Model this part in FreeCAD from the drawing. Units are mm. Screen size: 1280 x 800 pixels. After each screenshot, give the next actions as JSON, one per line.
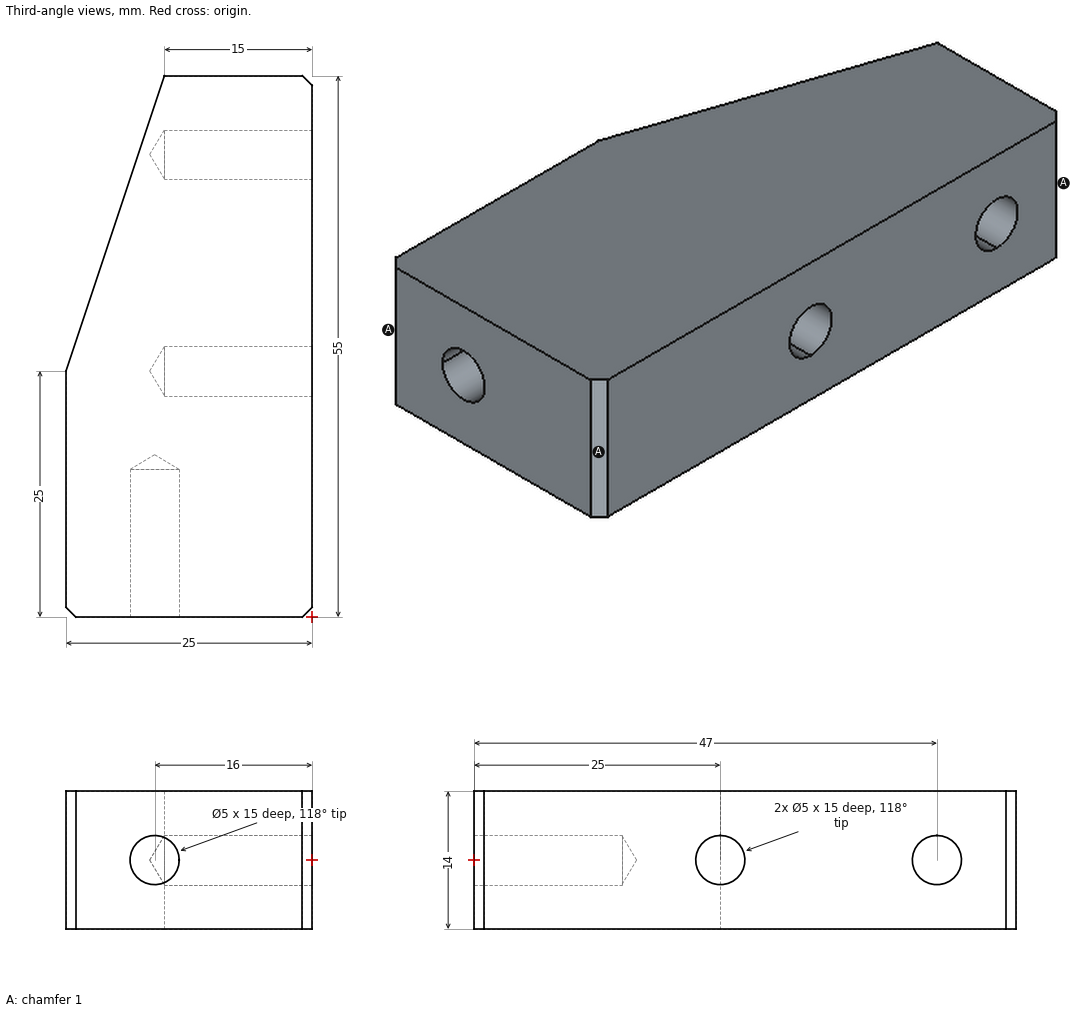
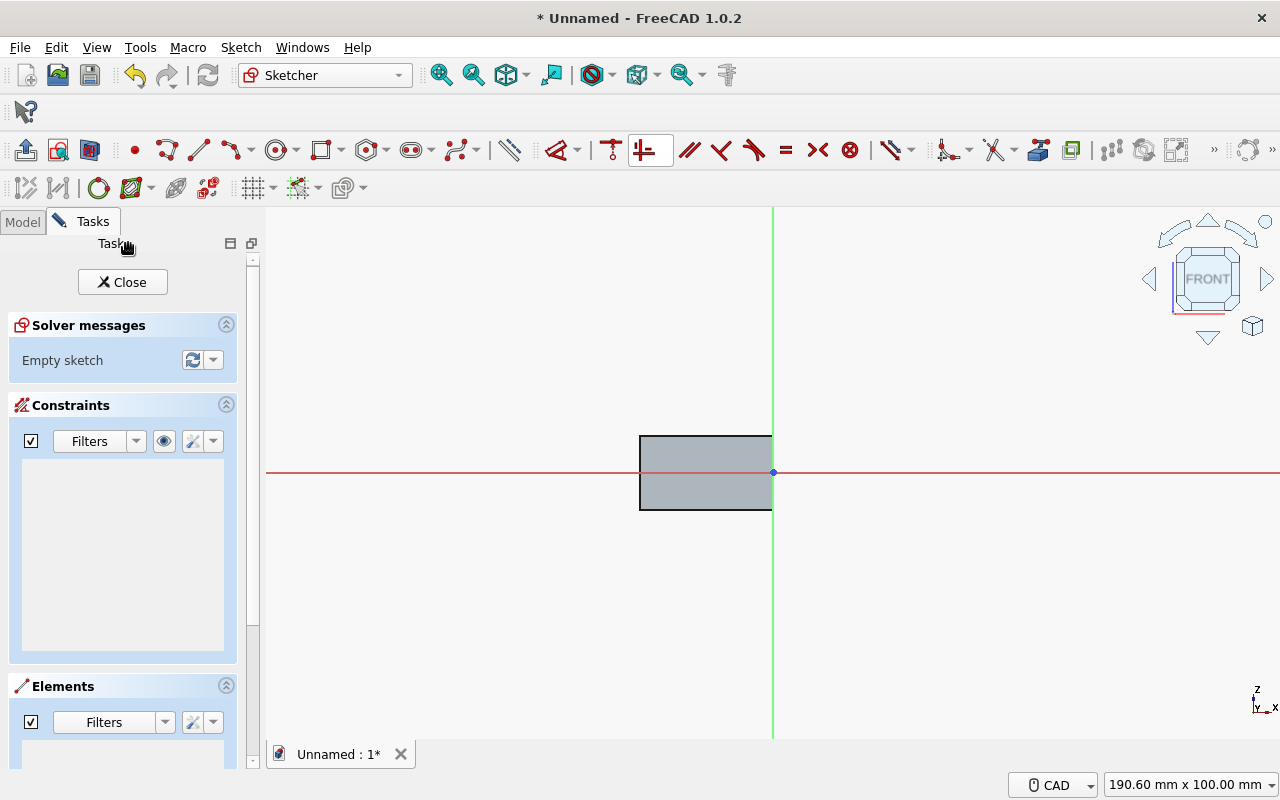
{"action": "scroll", "coordinate": [687, 473], "scroll_direction": "up", "scroll_amount": 13}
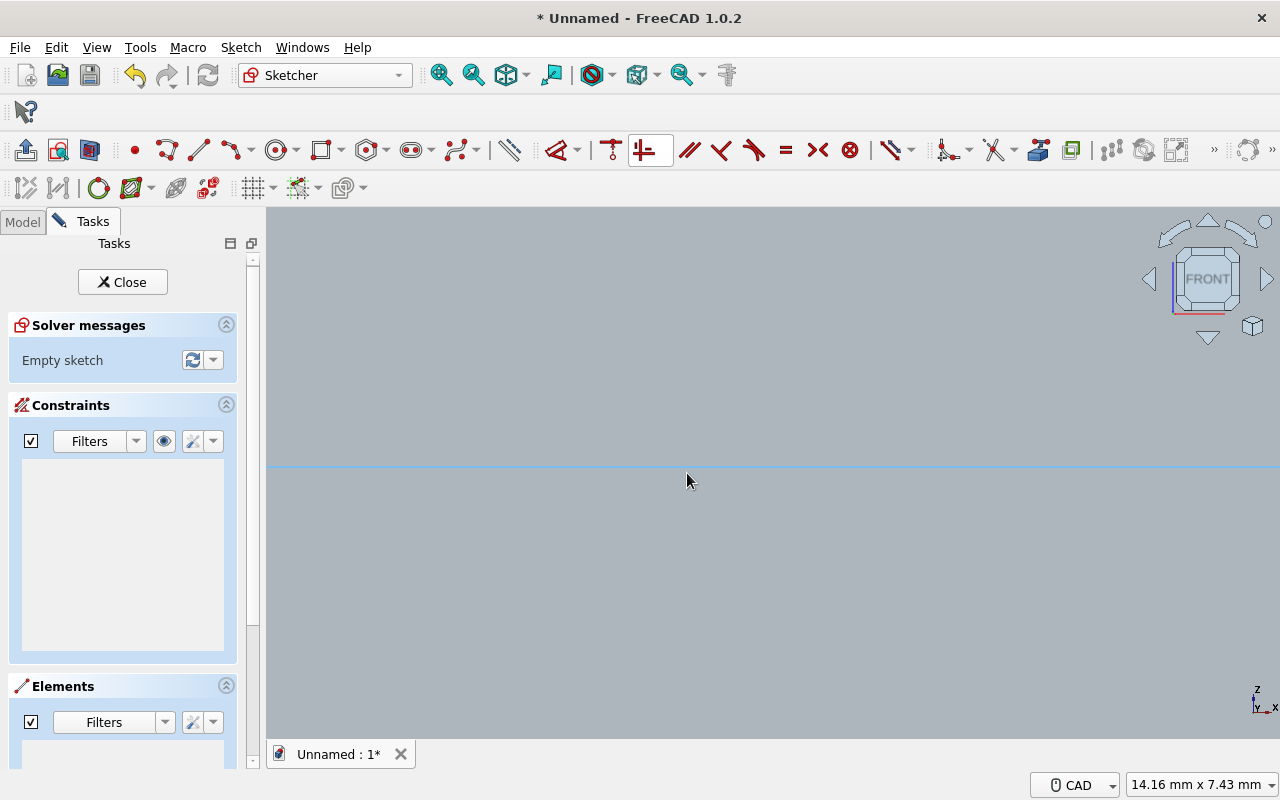
{"action": "key", "text": "g c"}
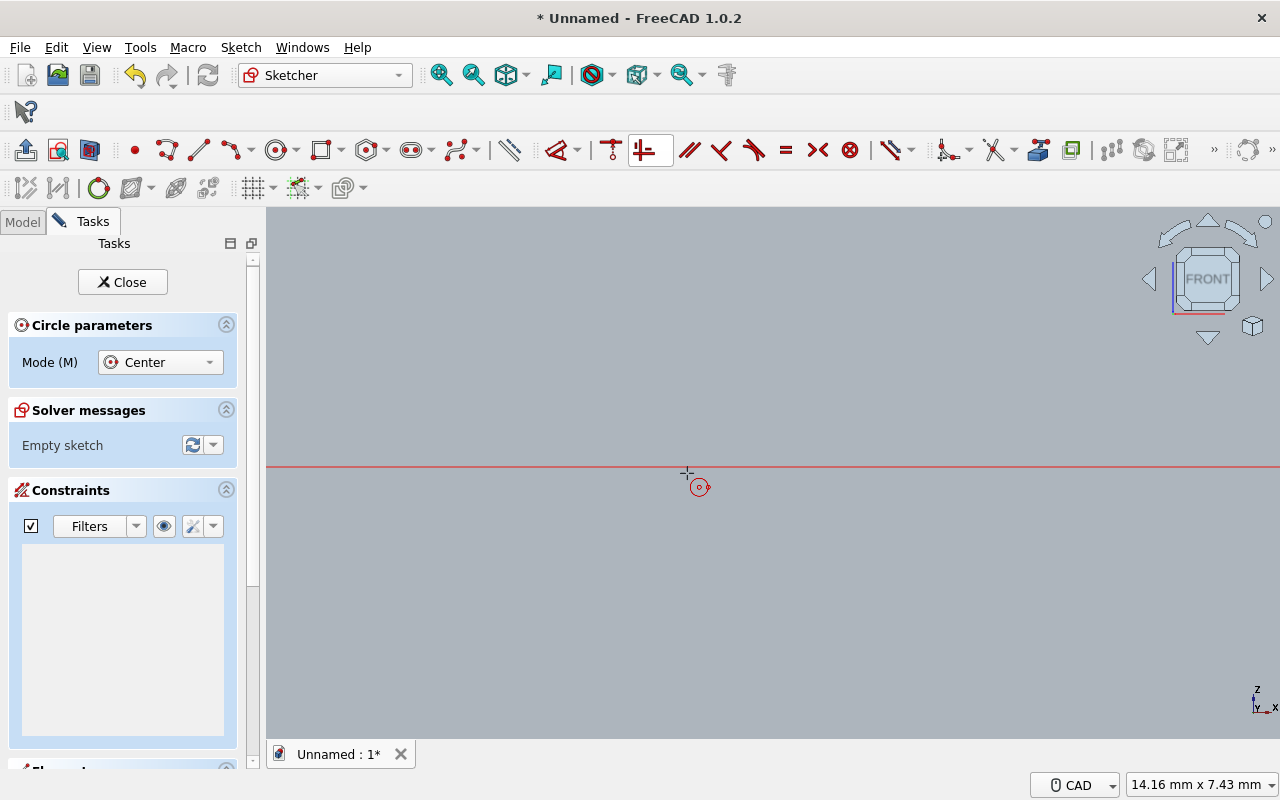
{"action": "left_click", "coordinate": [694, 467]}
{"action": "mouse_move", "coordinate": [820, 340]}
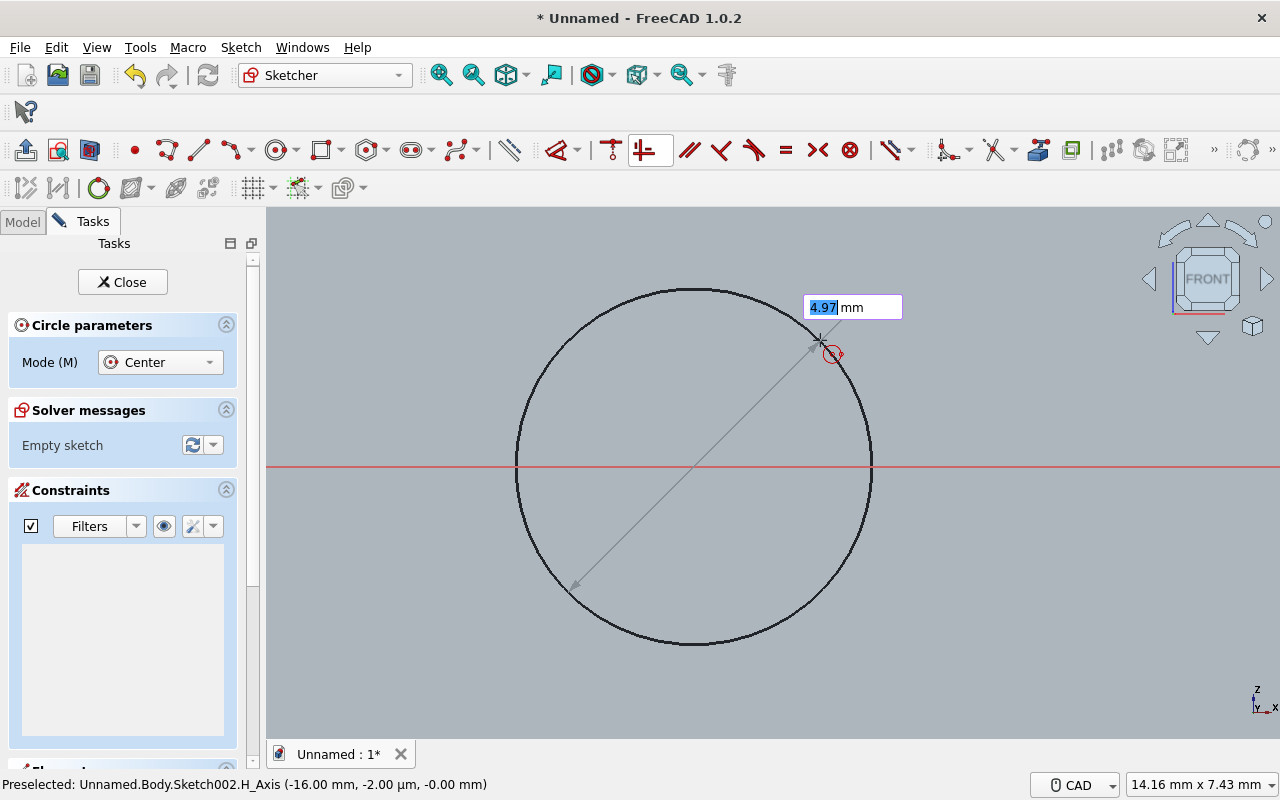
{"action": "type", "text": "5"}
{"action": "key", "text": "Return"}
{"action": "key", "text": "Escape"}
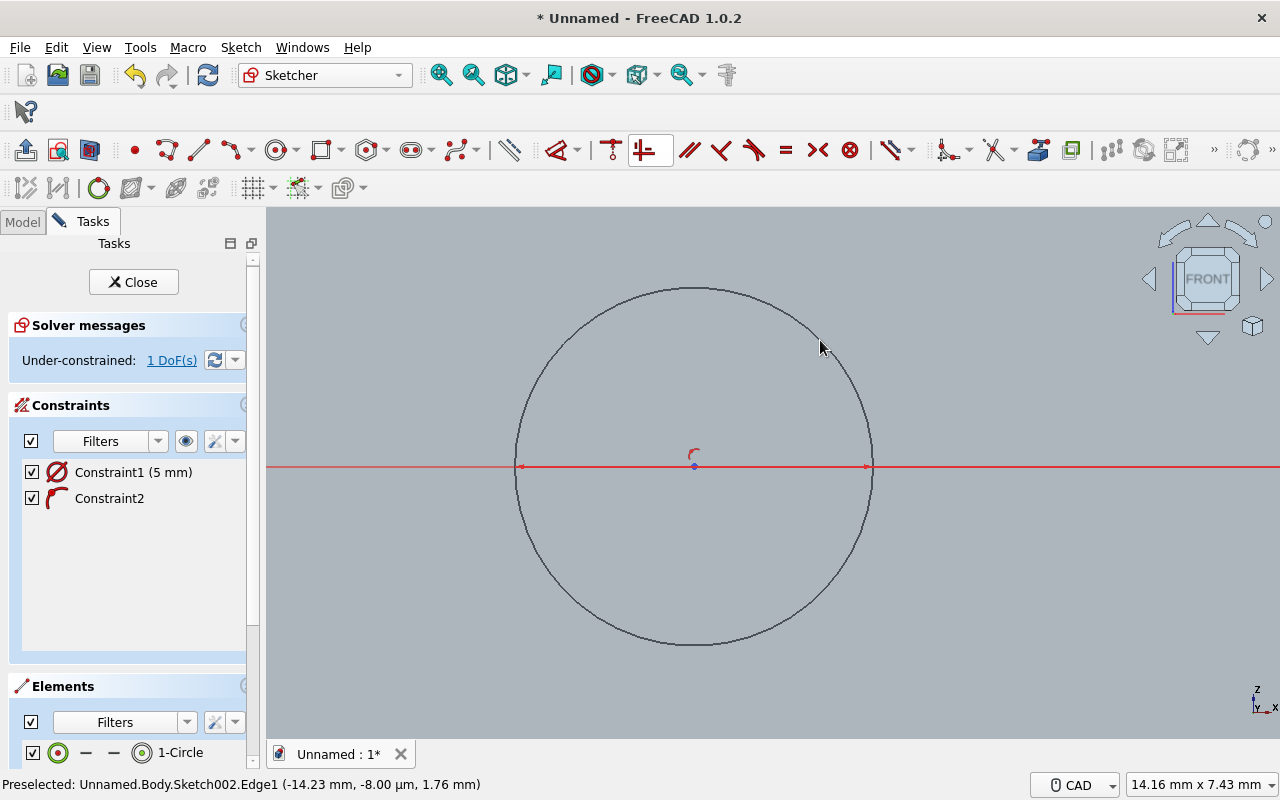
{"action": "left_click", "coordinate": [556, 150]}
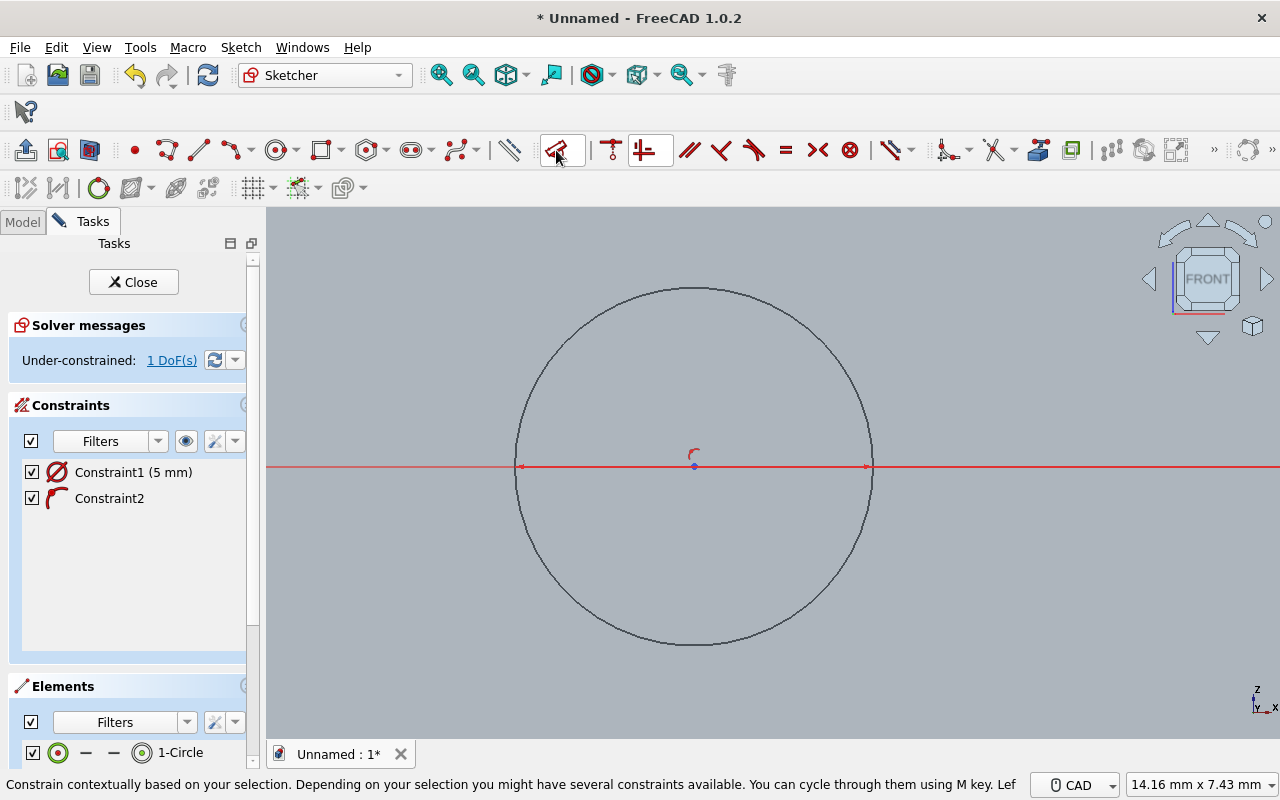
{"action": "left_click", "coordinate": [694, 467]}
{"action": "left_click", "coordinate": [905, 501]}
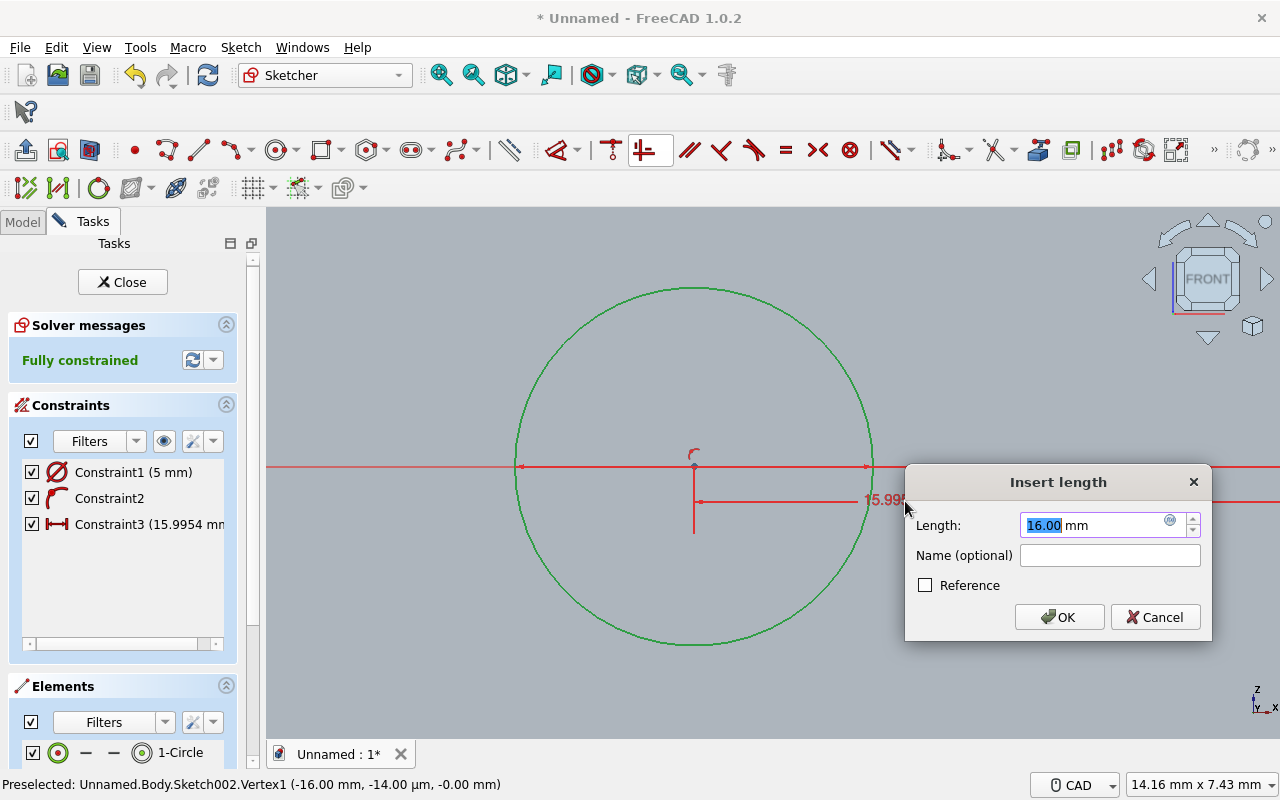
{"action": "type", "text": "16"}
{"action": "key", "text": "Return"}
{"action": "key", "text": "Escape"}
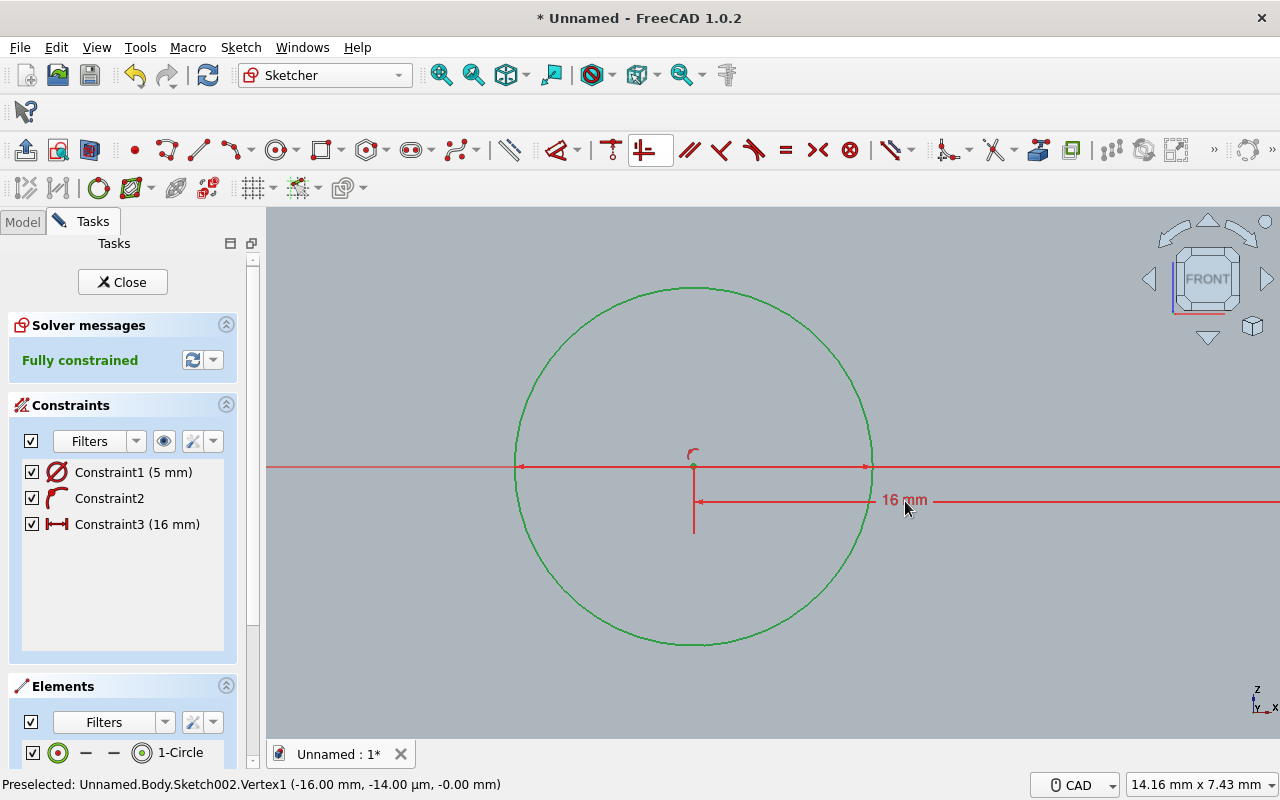
{"action": "left_click", "coordinate": [123, 282]}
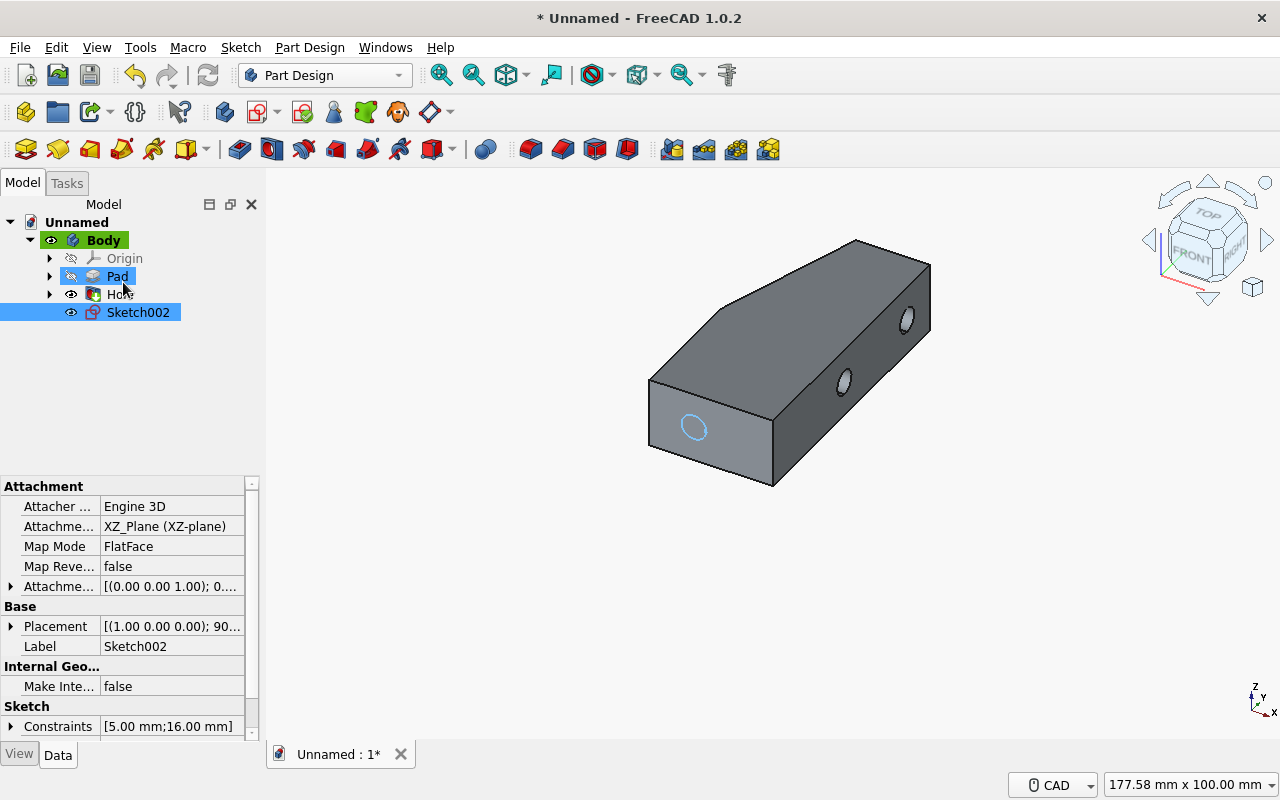
{"action": "left_click", "coordinate": [272, 150]}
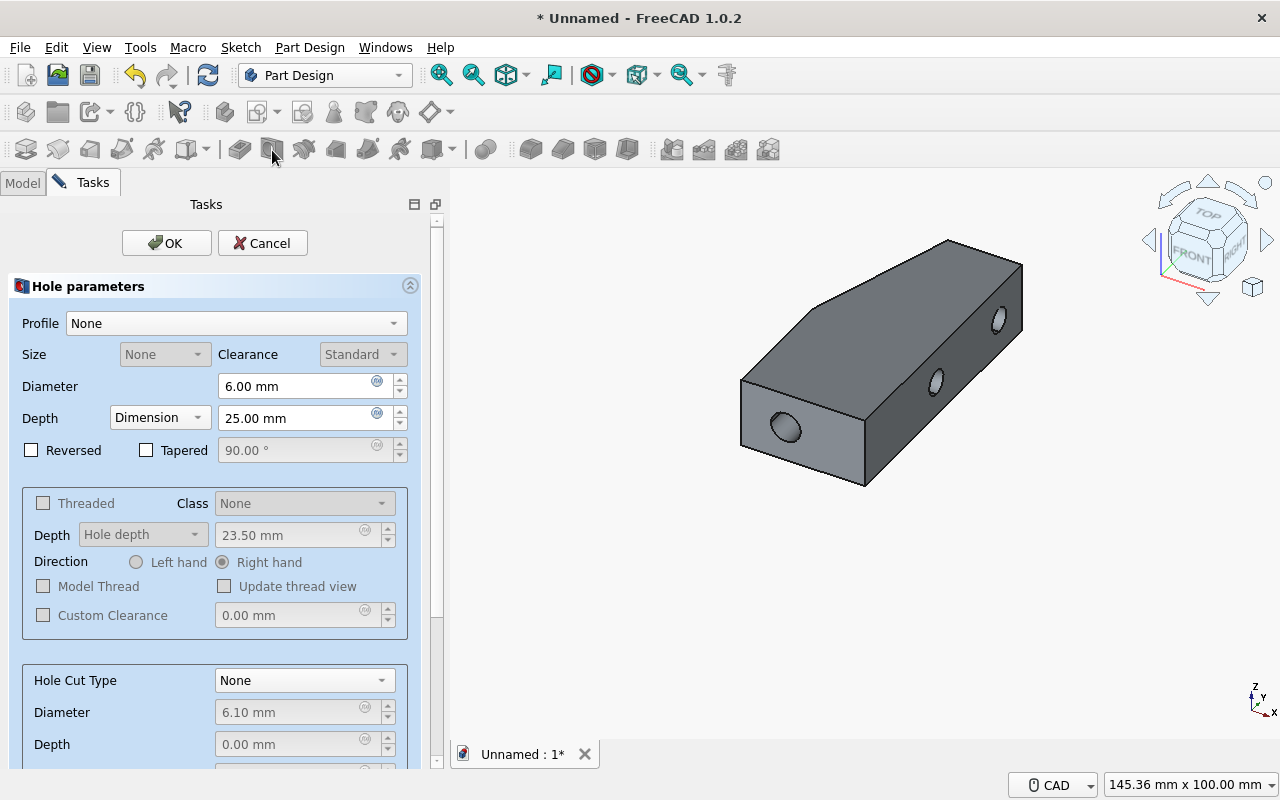
{"action": "triple_click", "coordinate": [305, 386]}